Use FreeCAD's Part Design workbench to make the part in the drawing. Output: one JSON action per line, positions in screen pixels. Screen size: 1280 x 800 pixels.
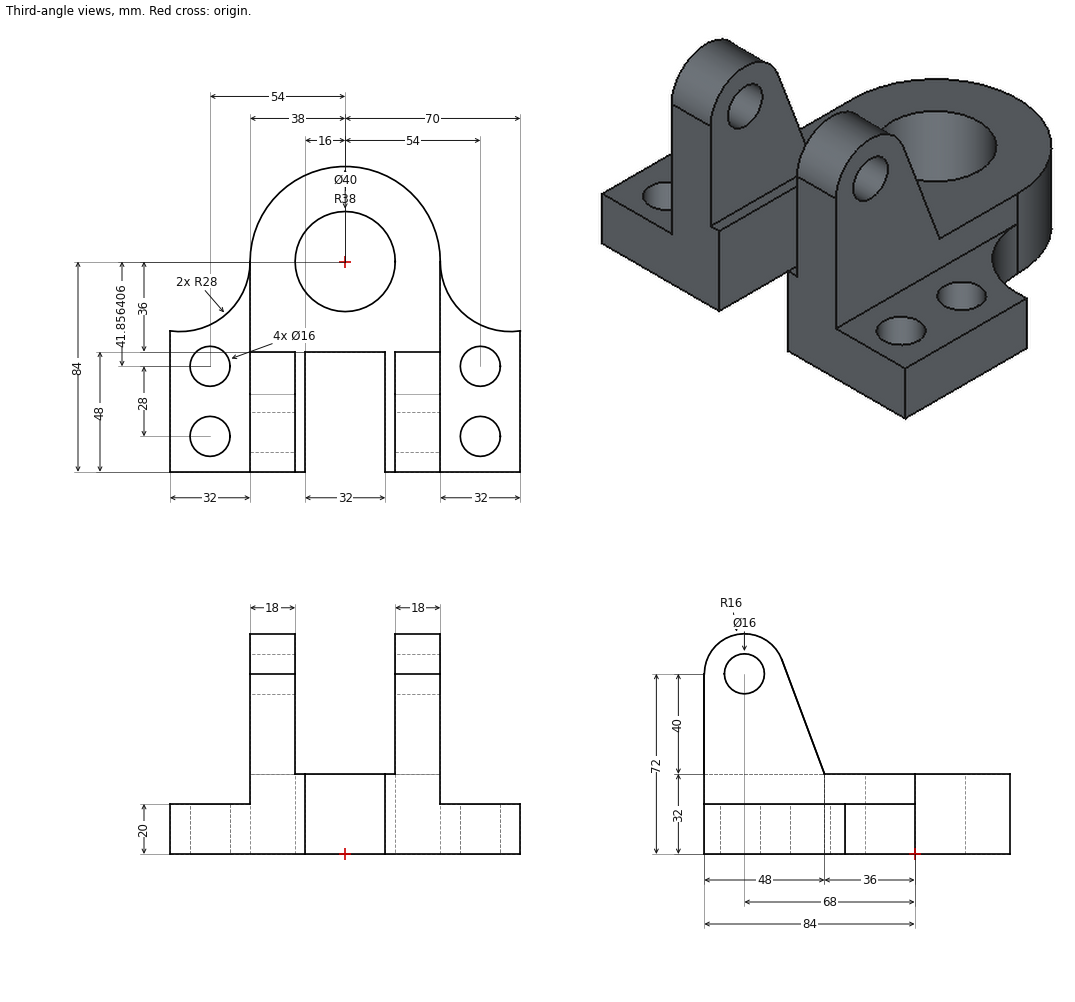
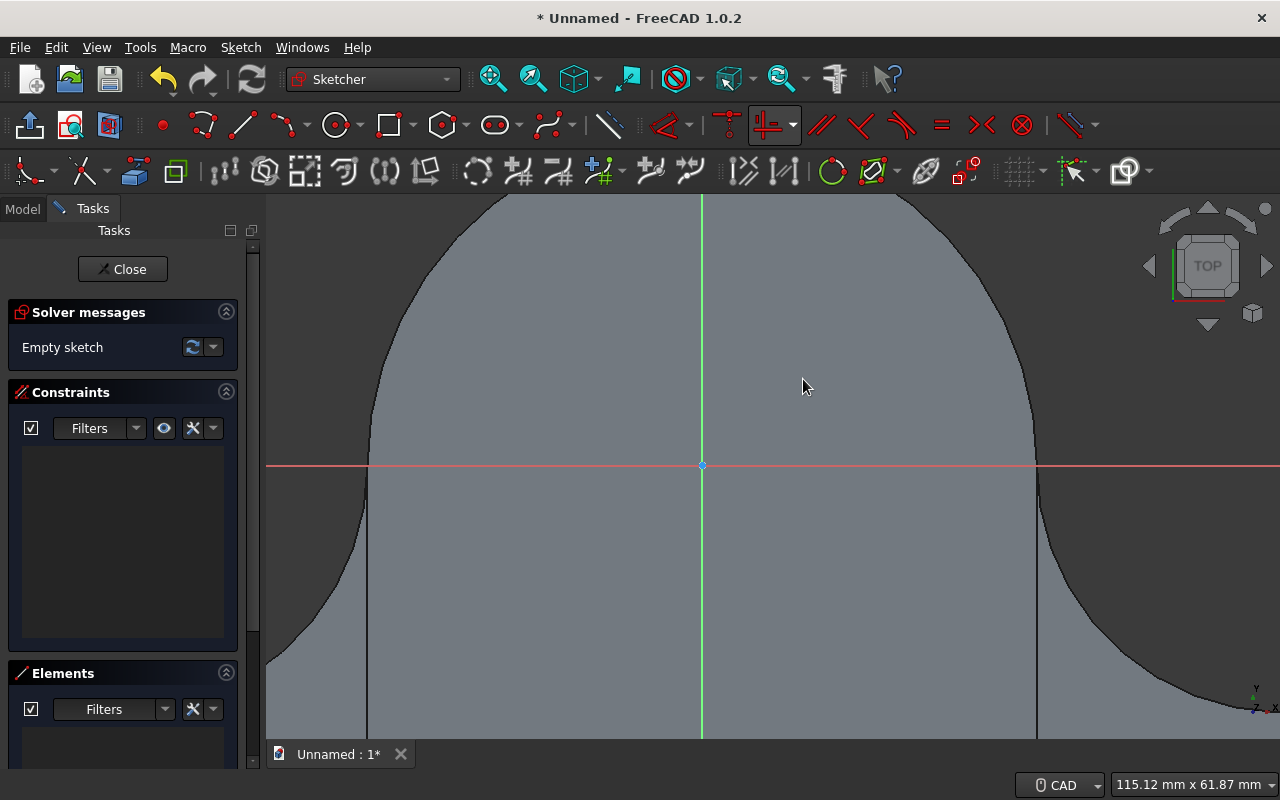
{"action": "left_click", "coordinate": [336, 126]}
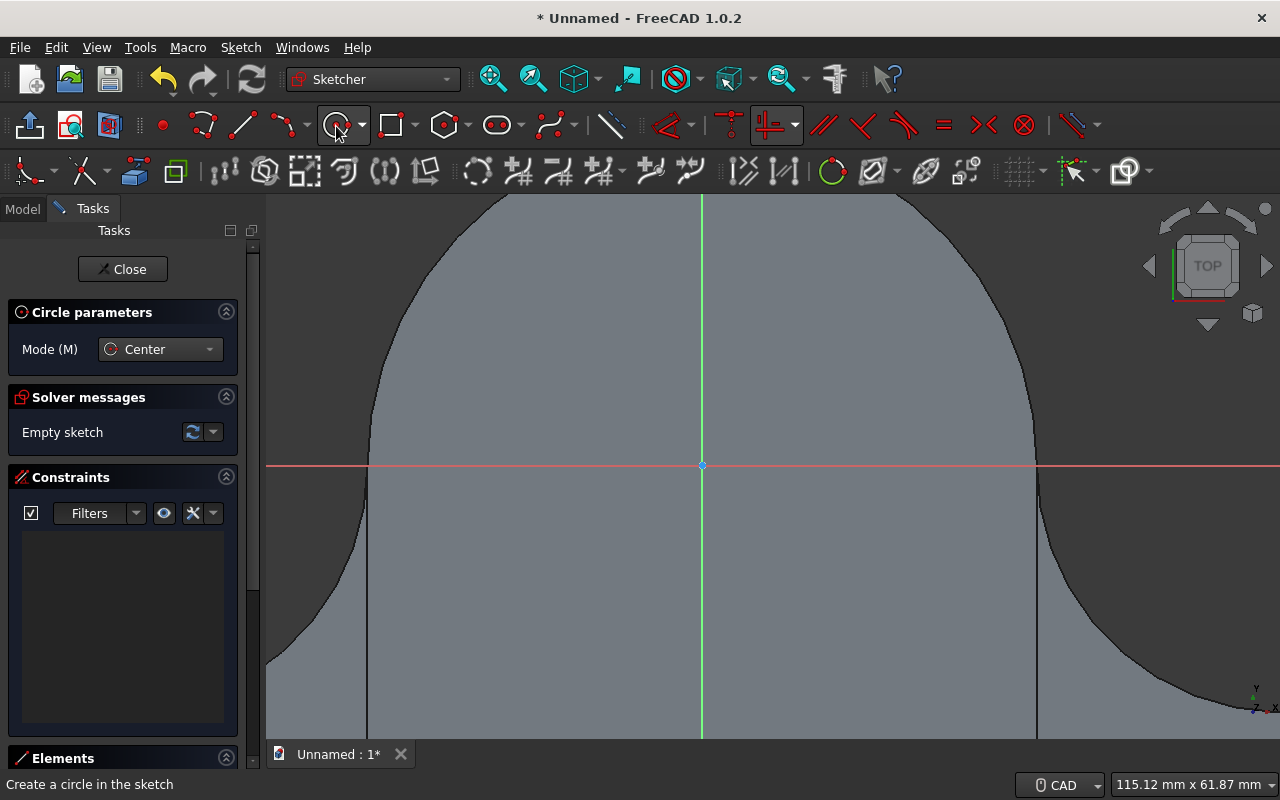
{"action": "left_click", "coordinate": [702, 466]}
{"action": "left_click", "coordinate": [827, 341]}
{"action": "key", "text": "Escape"}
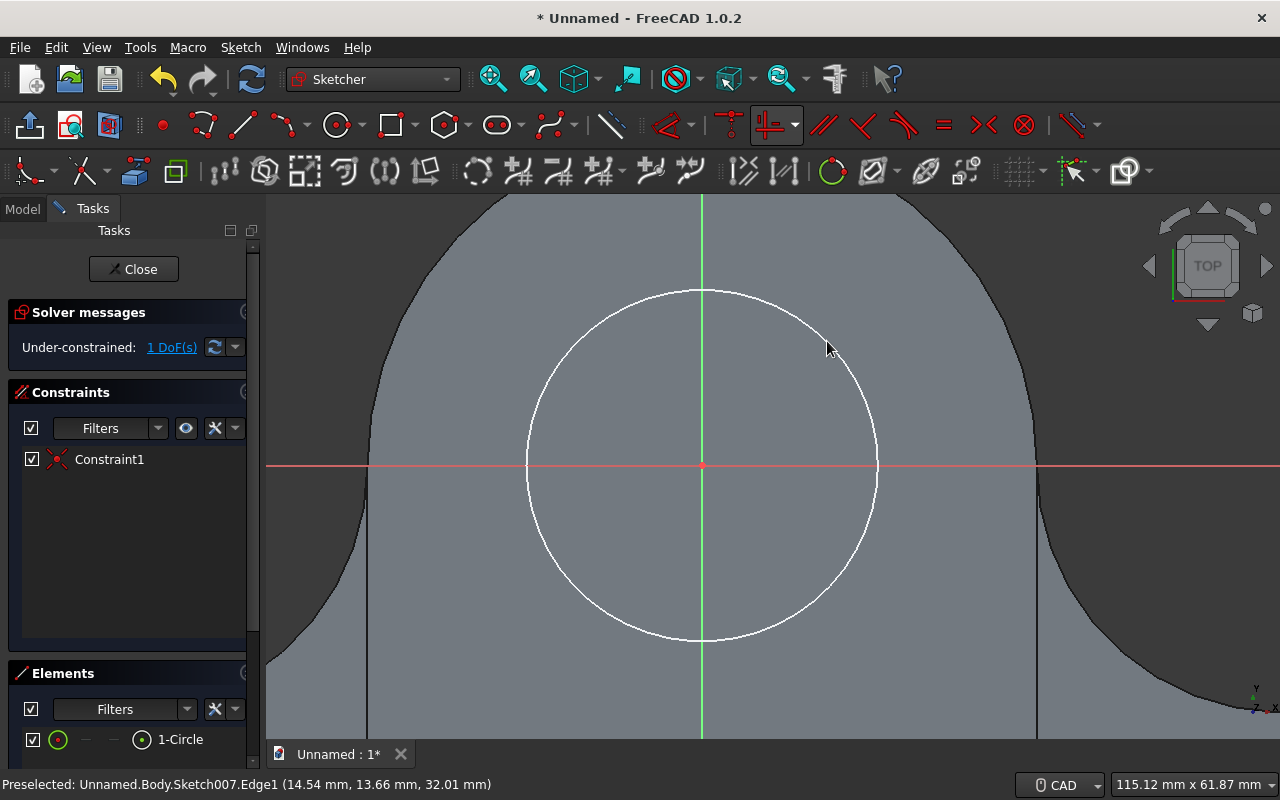
{"action": "left_click", "coordinate": [666, 126]}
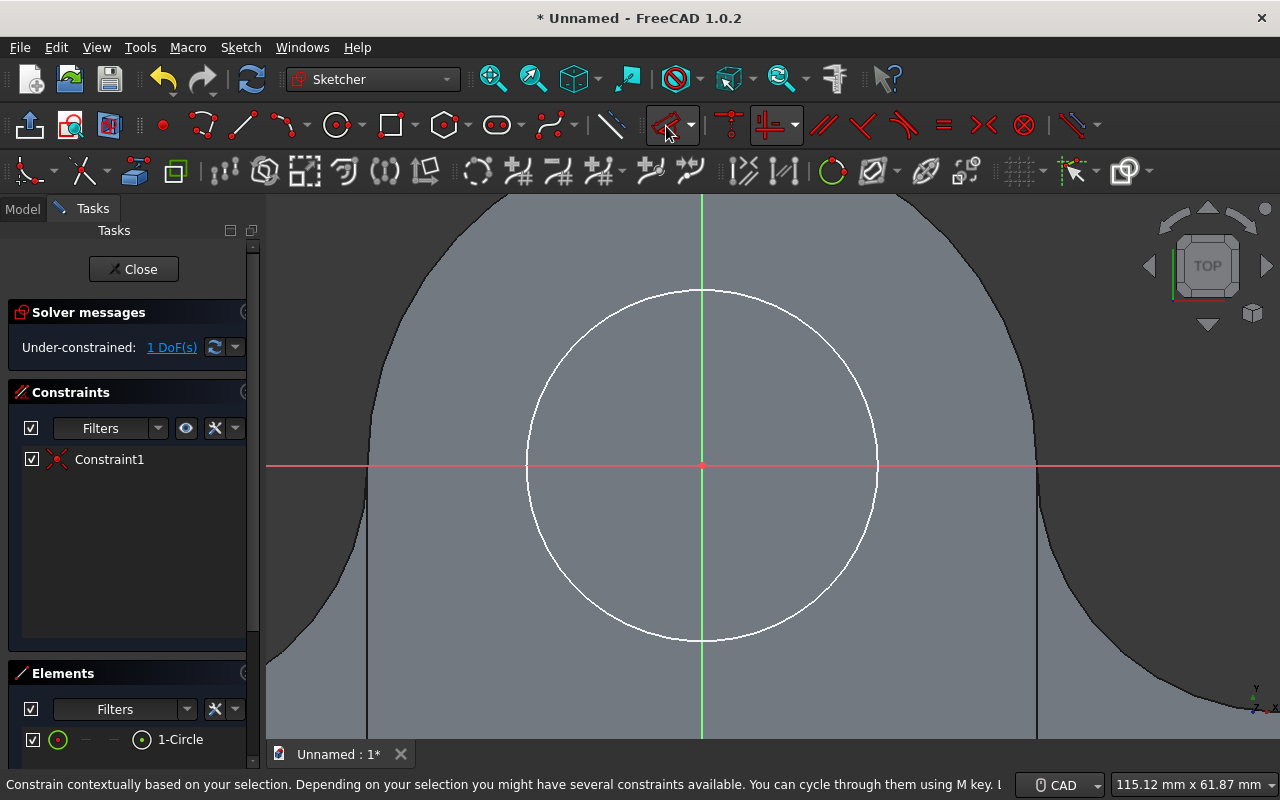
{"action": "left_click", "coordinate": [826, 341]}
{"action": "left_click", "coordinate": [849, 318]}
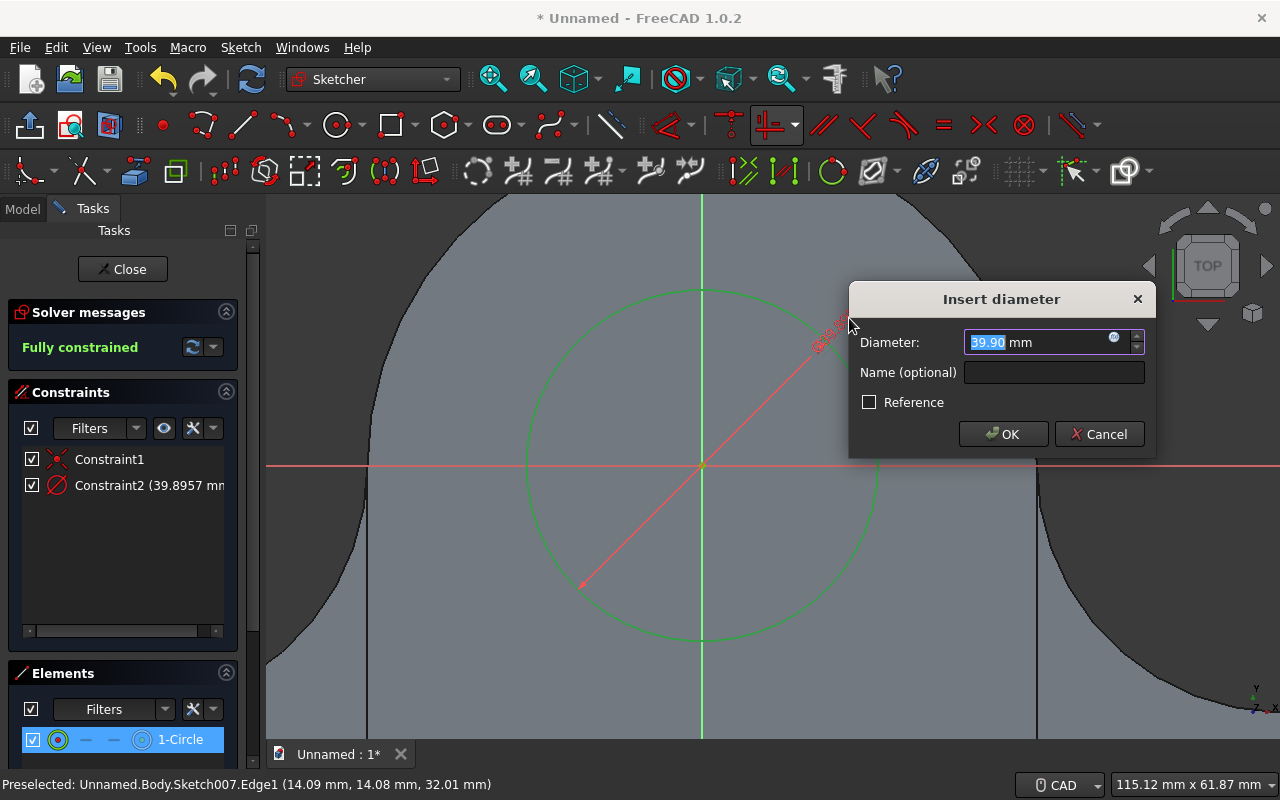
{"action": "type", "text": "40"}
{"action": "key", "text": "Return"}
{"action": "key", "text": "Escape"}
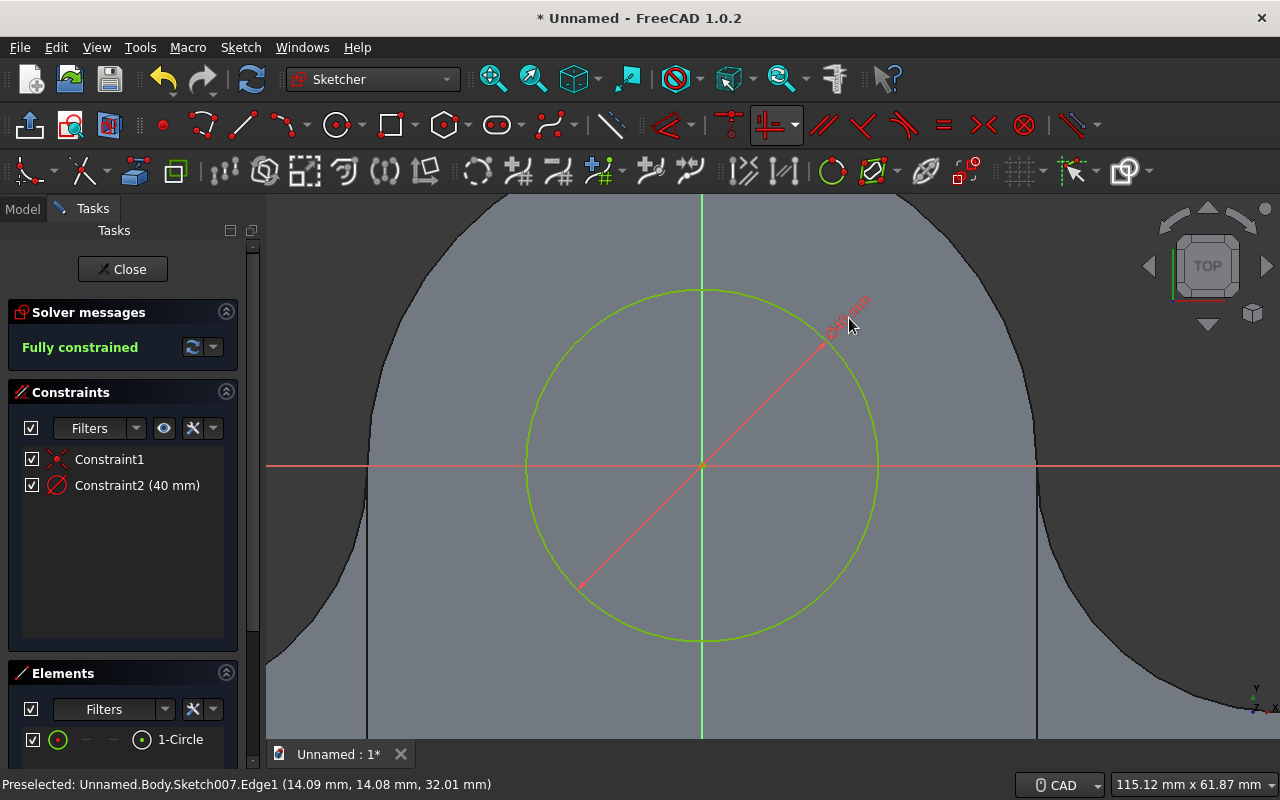
{"action": "left_click", "coordinate": [123, 269]}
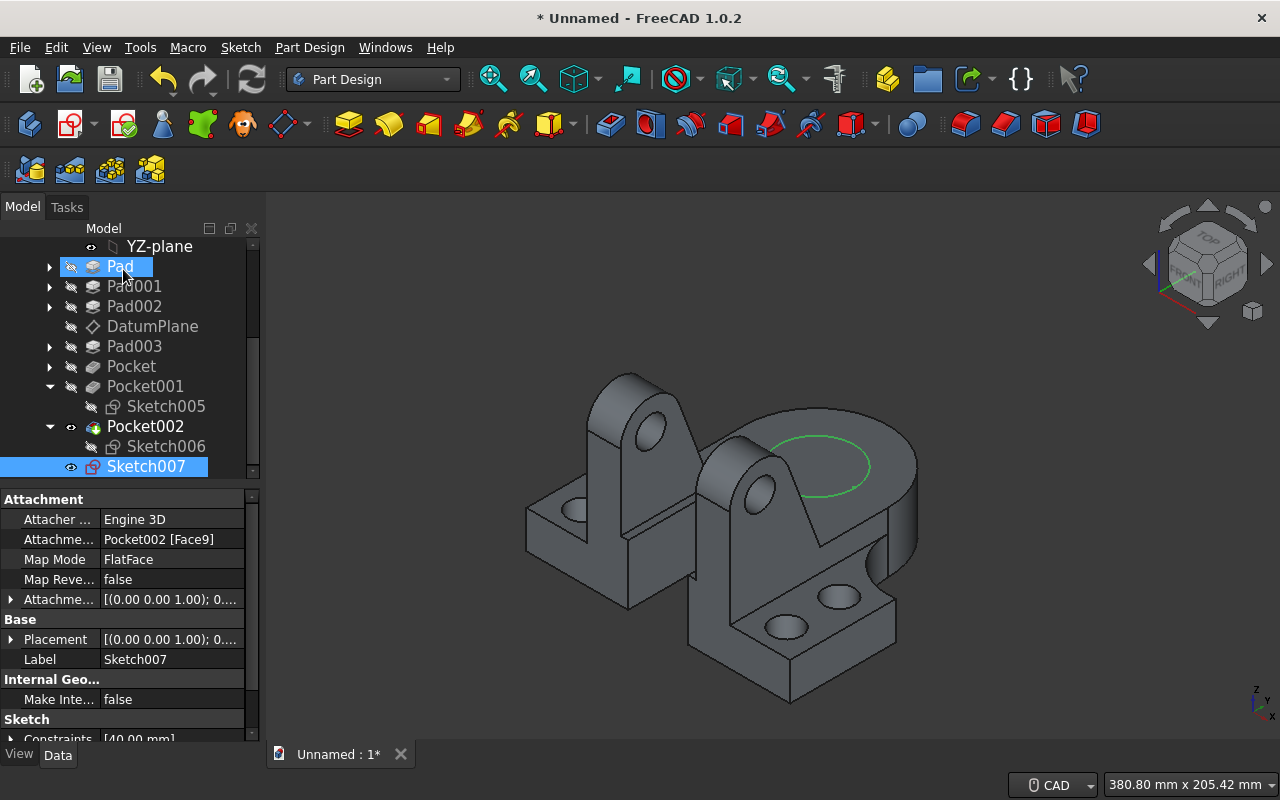
{"action": "left_click", "coordinate": [612, 124]}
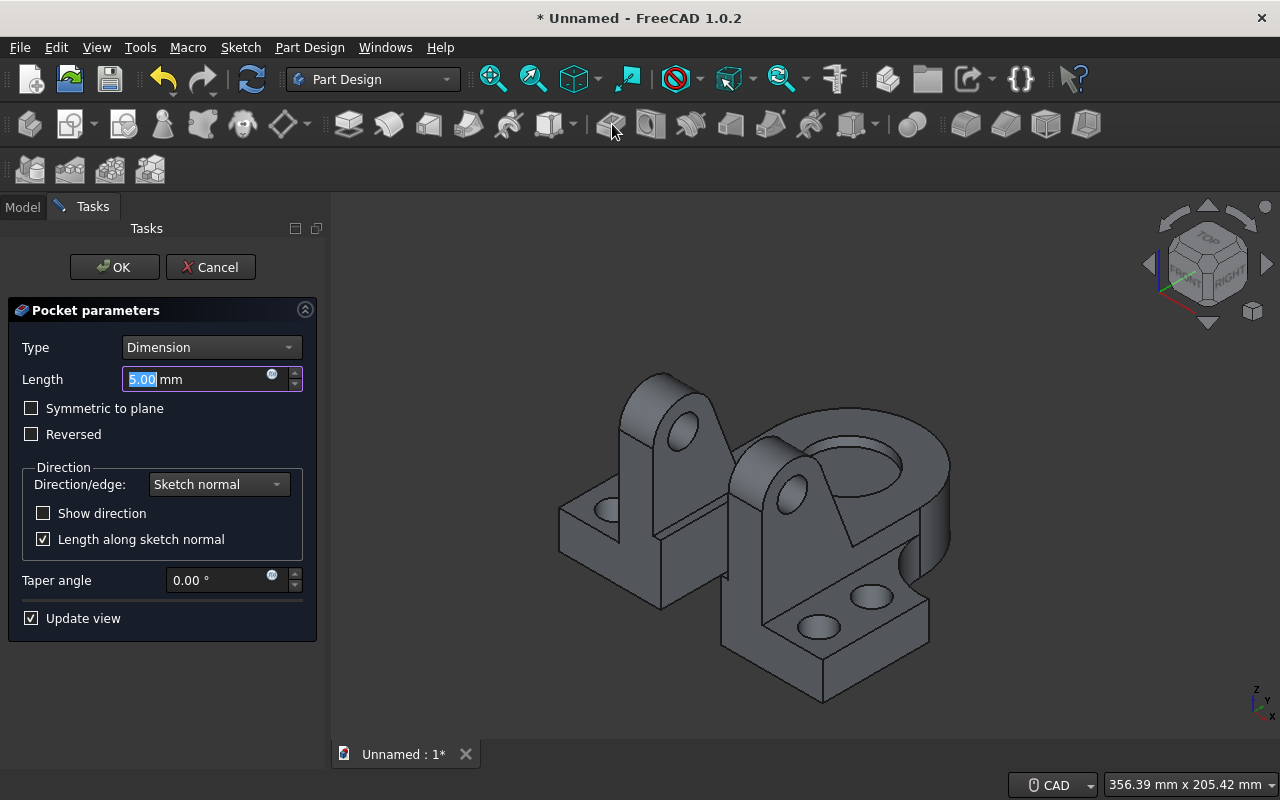
{"action": "left_click", "coordinate": [212, 348]}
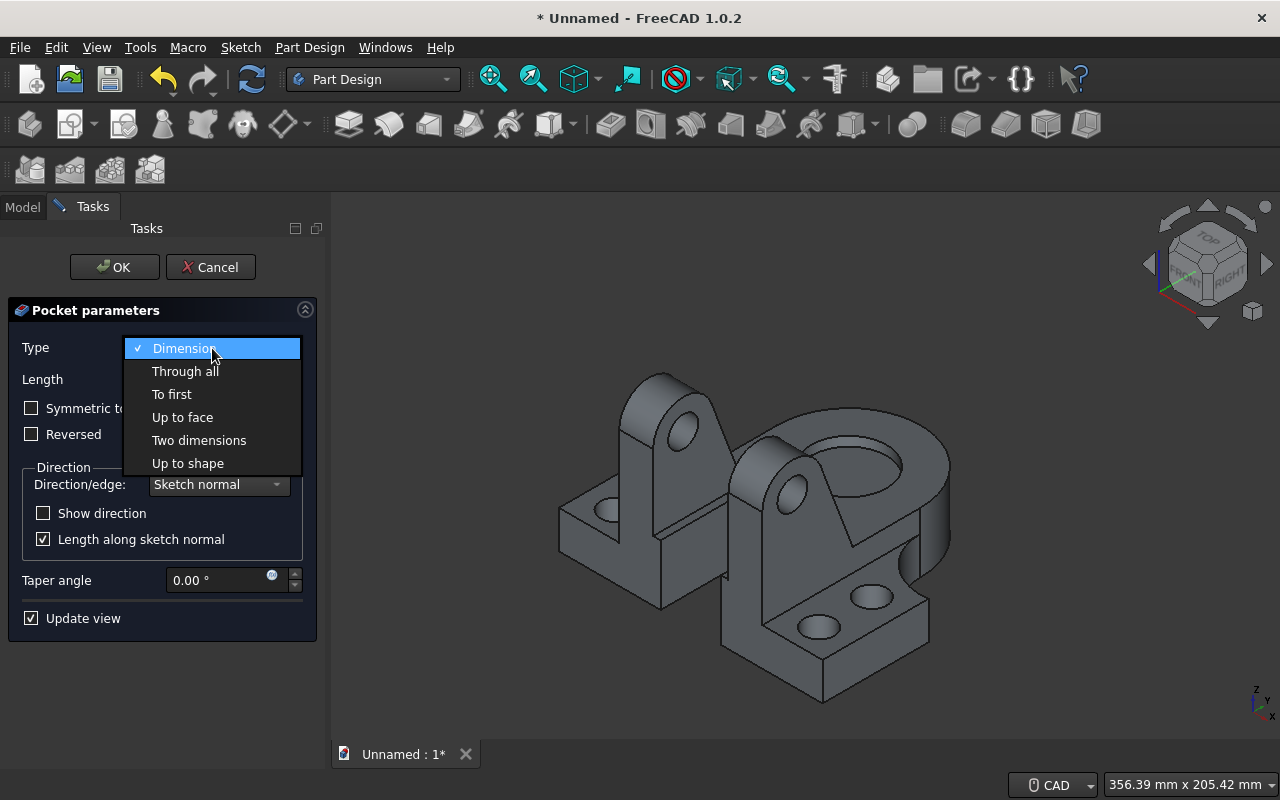
{"action": "left_click", "coordinate": [212, 372]}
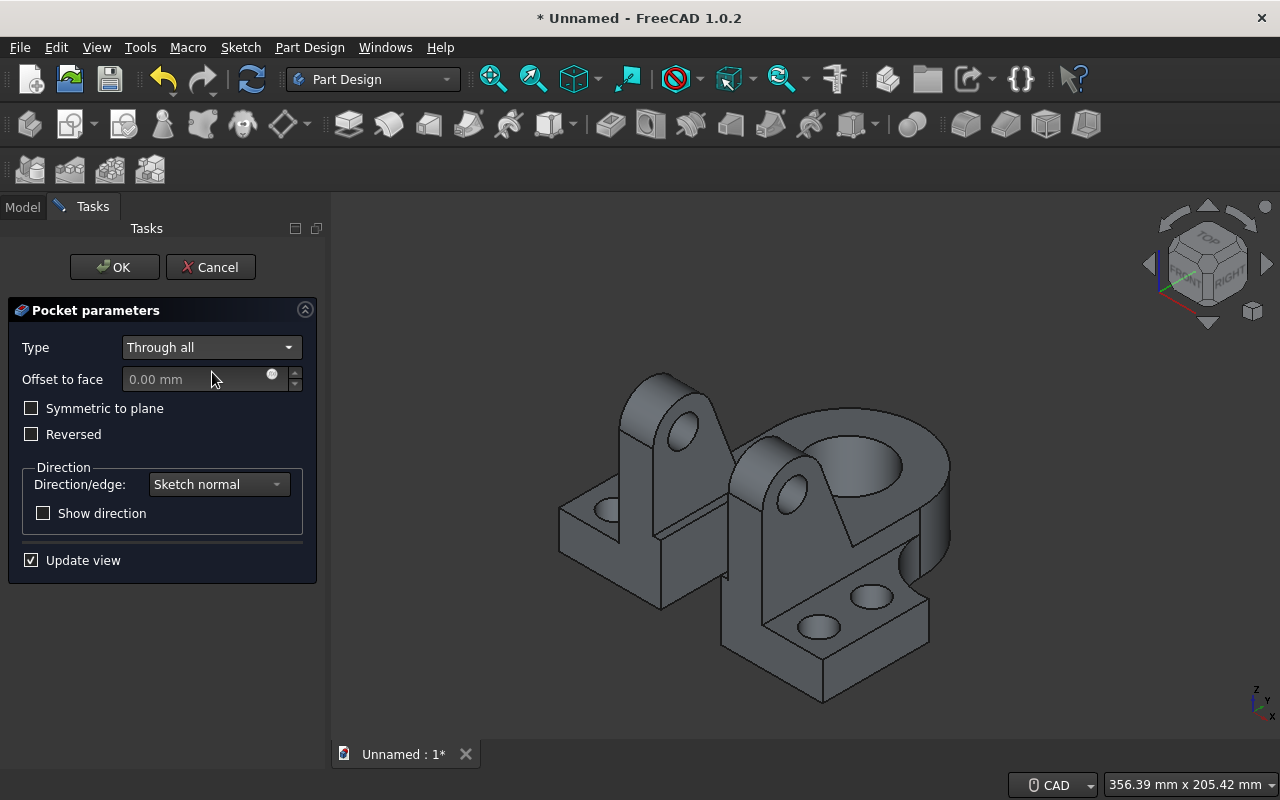
{"action": "left_click", "coordinate": [115, 267]}